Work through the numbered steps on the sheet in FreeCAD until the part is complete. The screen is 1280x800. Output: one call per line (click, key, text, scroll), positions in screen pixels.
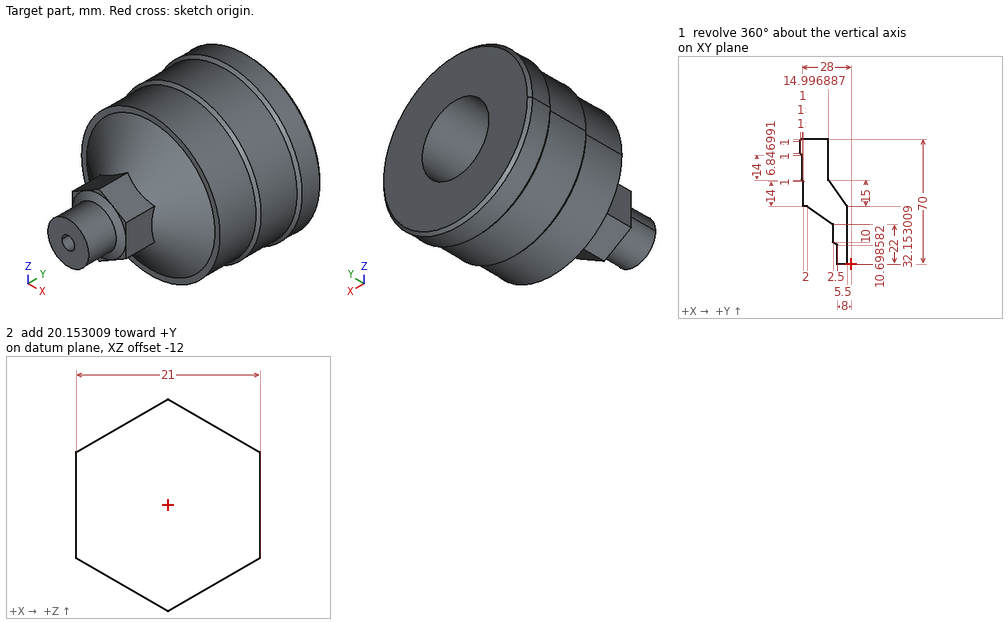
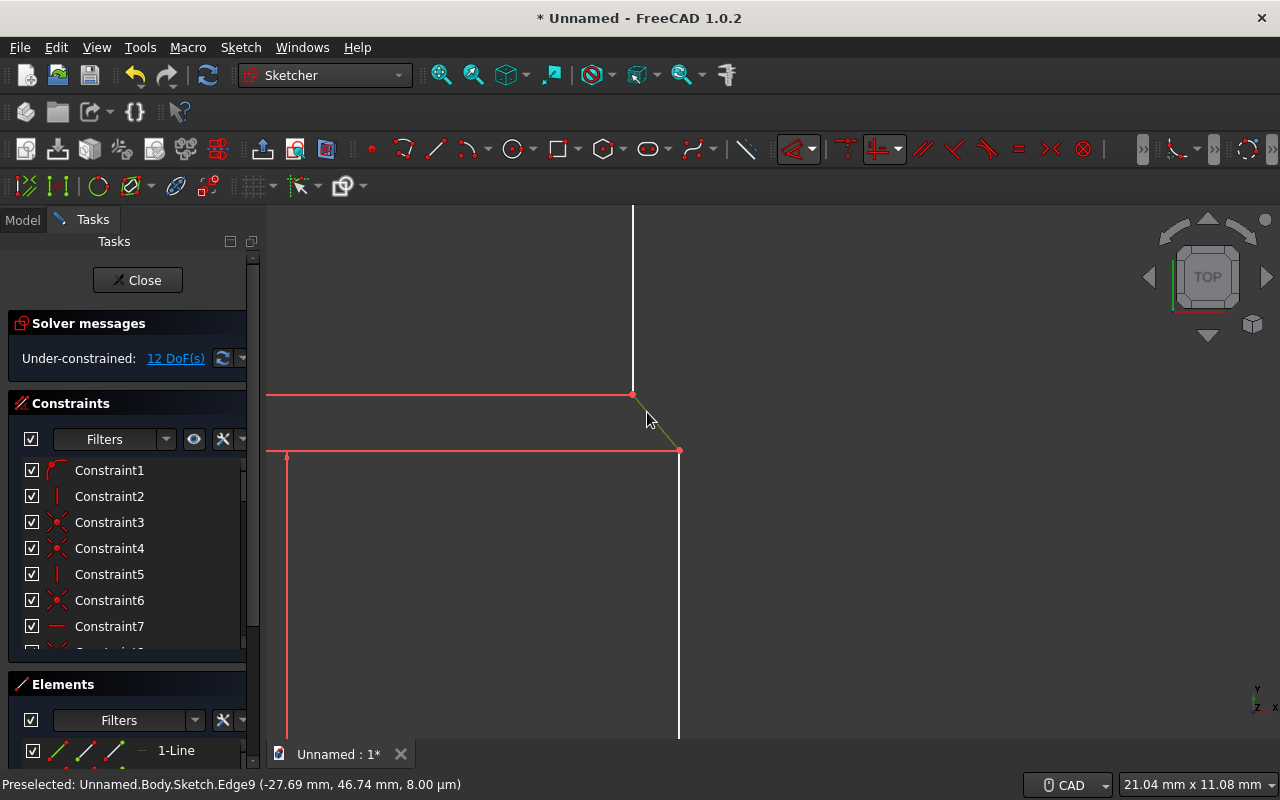
key(l)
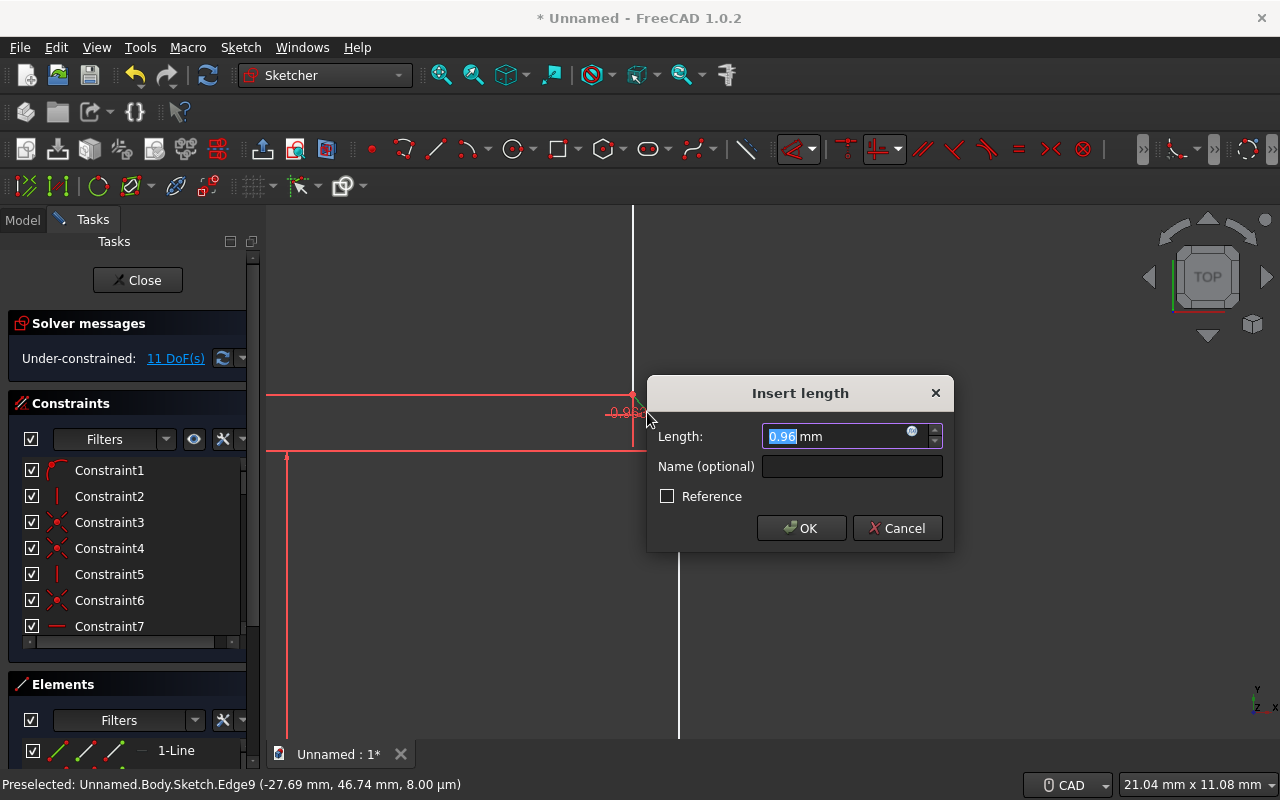
text(1)
key(Return)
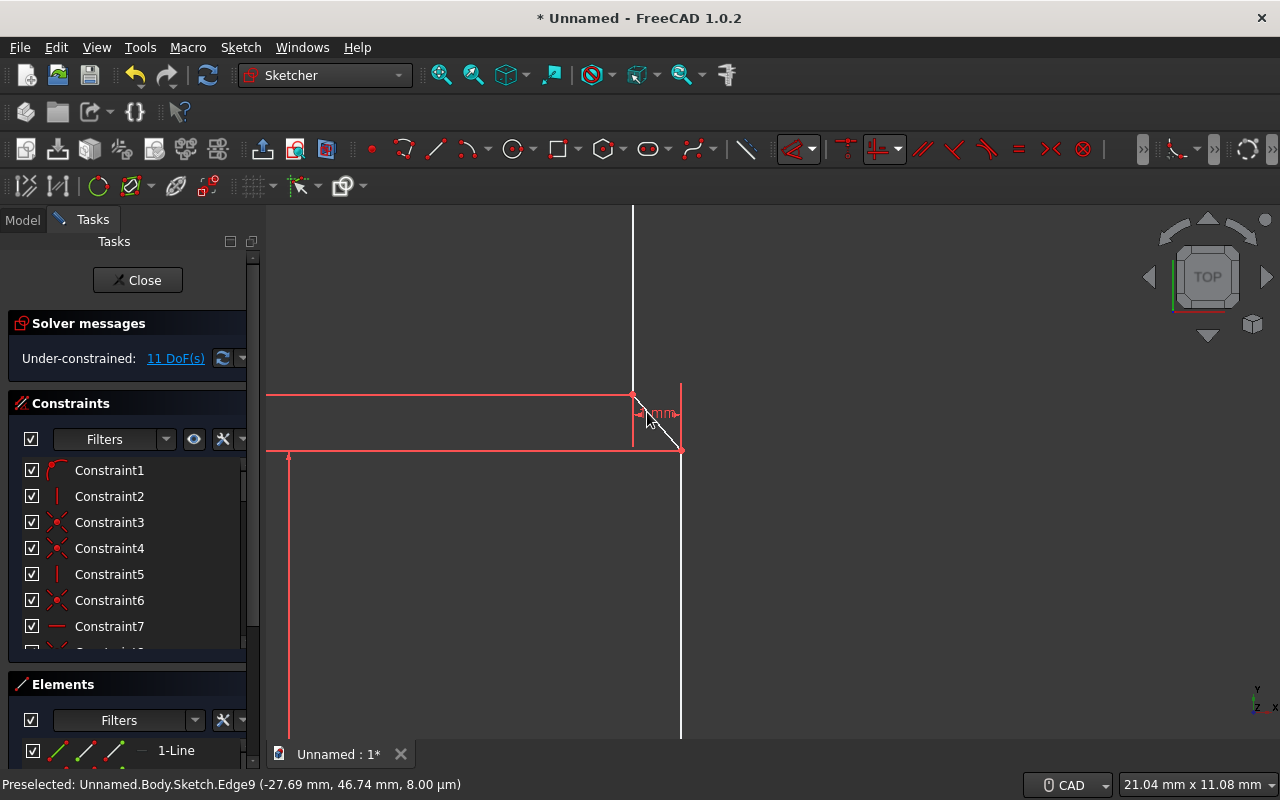
click(667, 434)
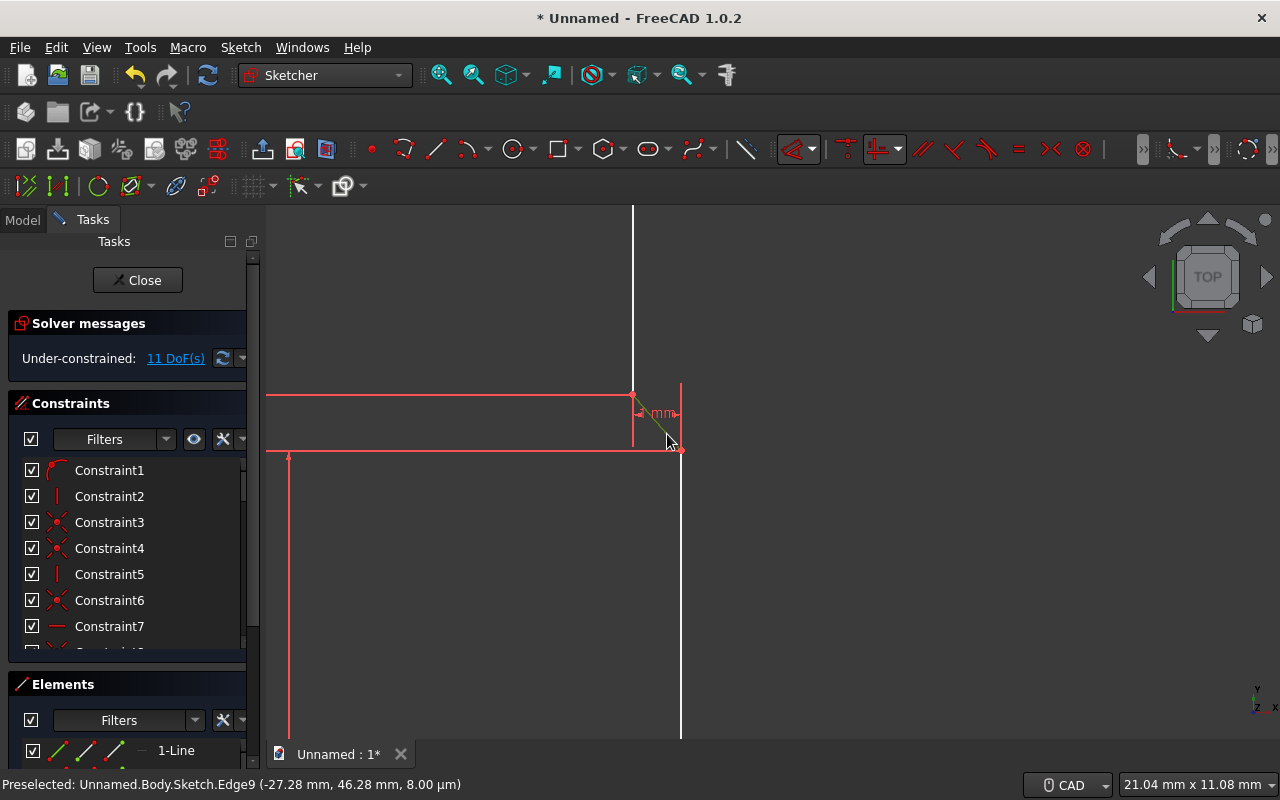
click(814, 150)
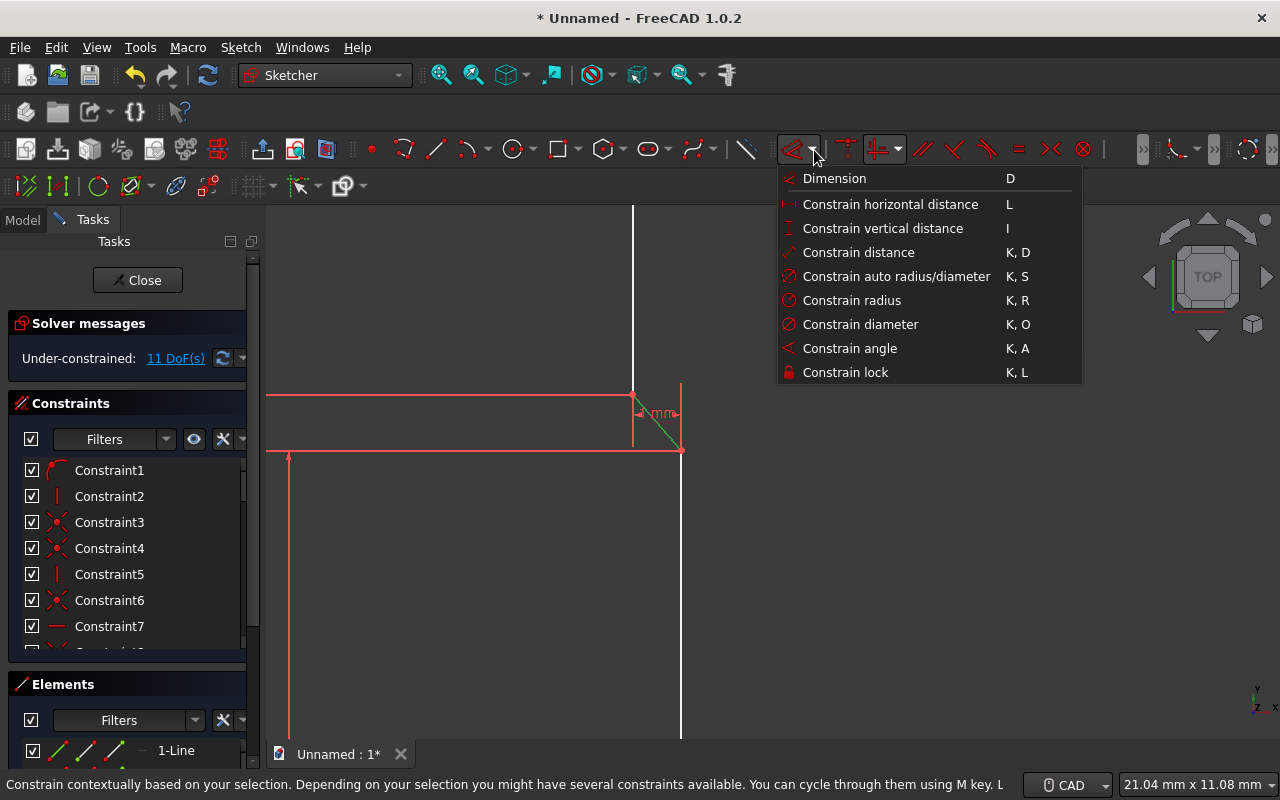
click(930, 228)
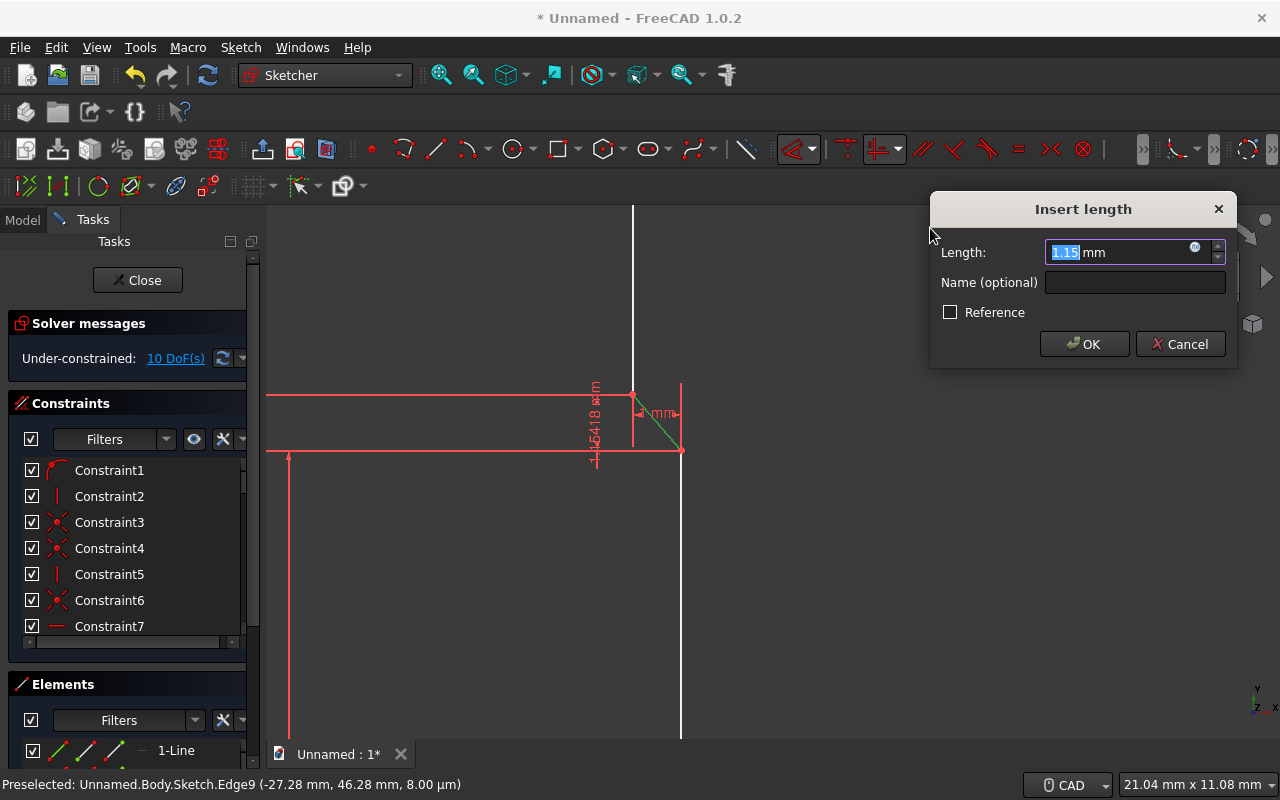
text(1)
key(Return)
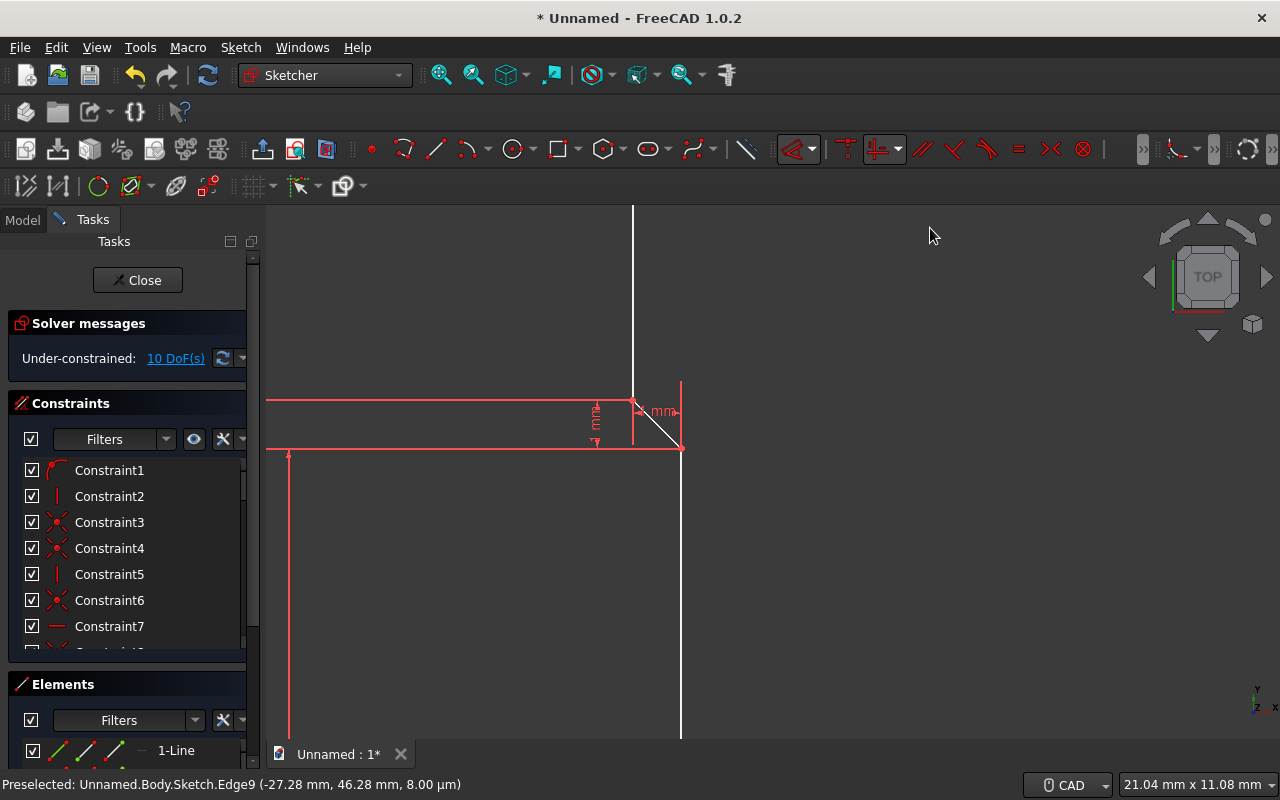
scroll(647, 422, down, 12)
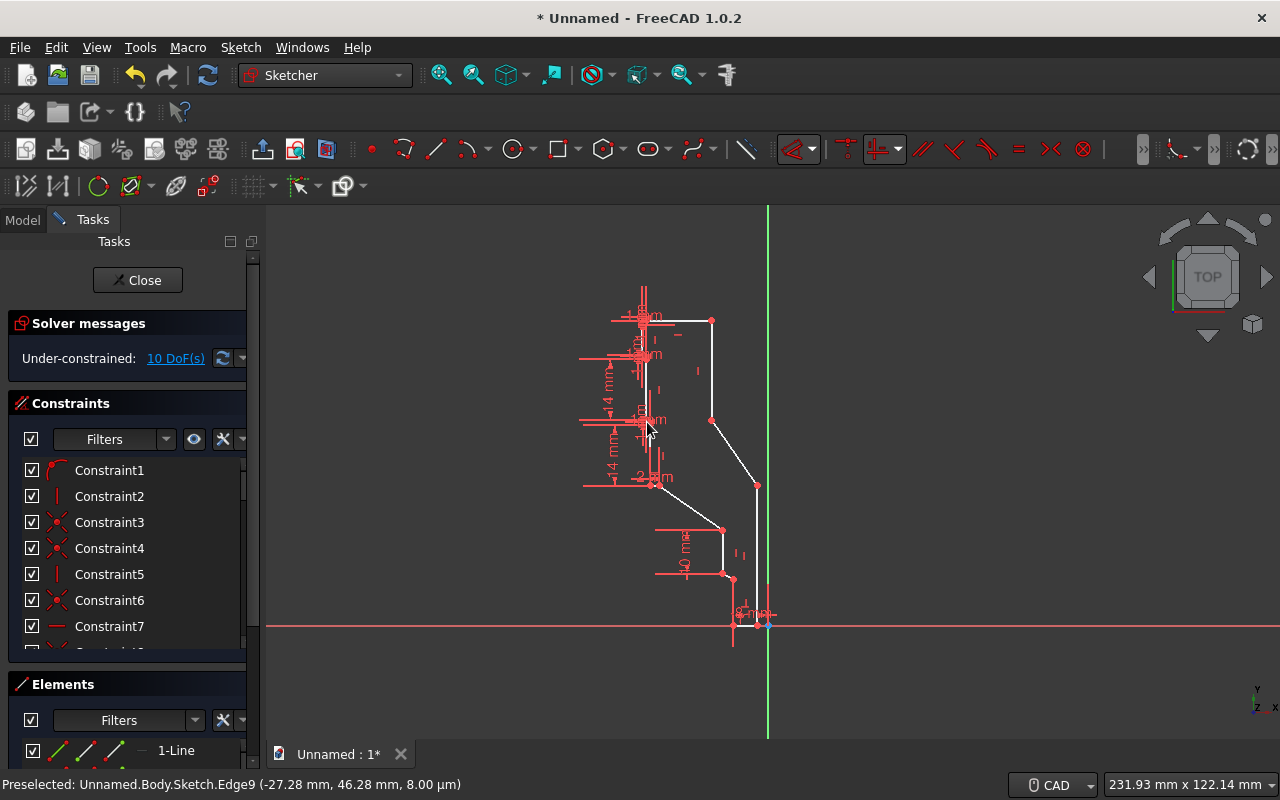
scroll(741, 626, up, 4)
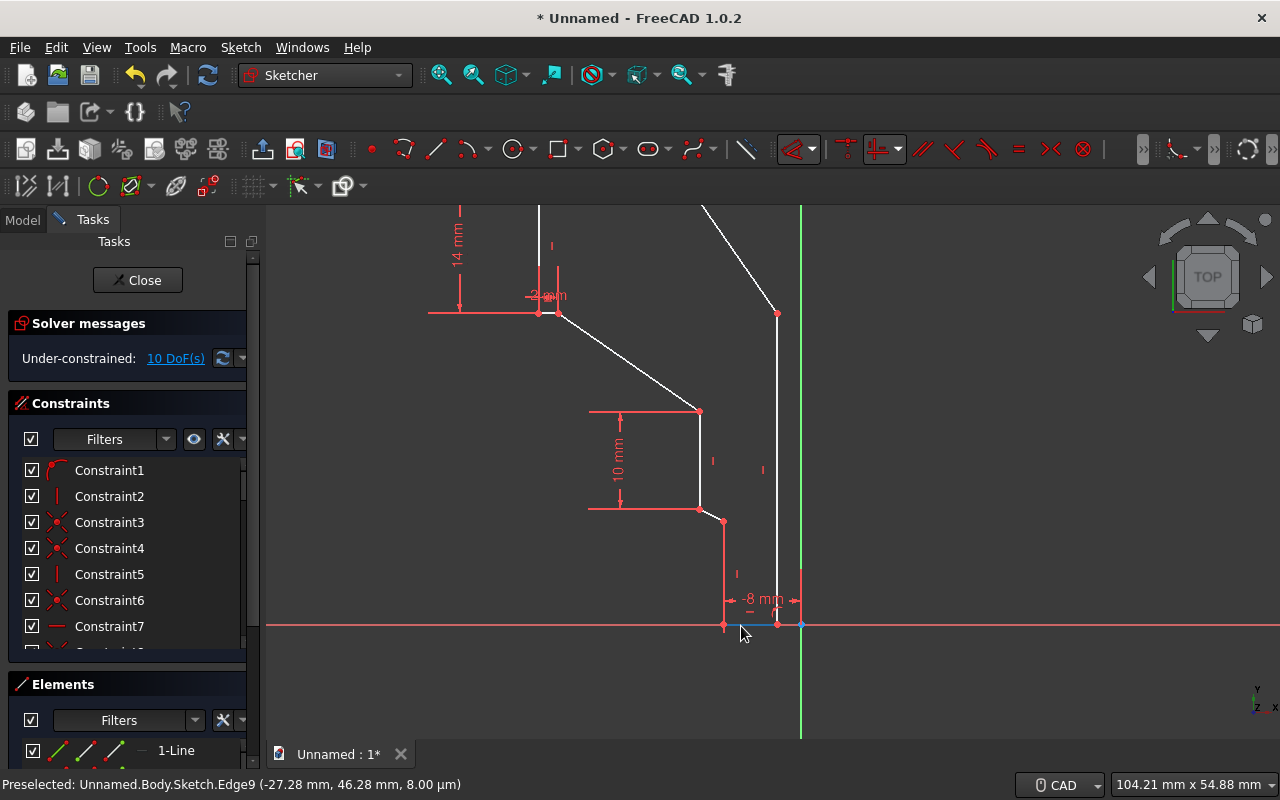
click(740, 625)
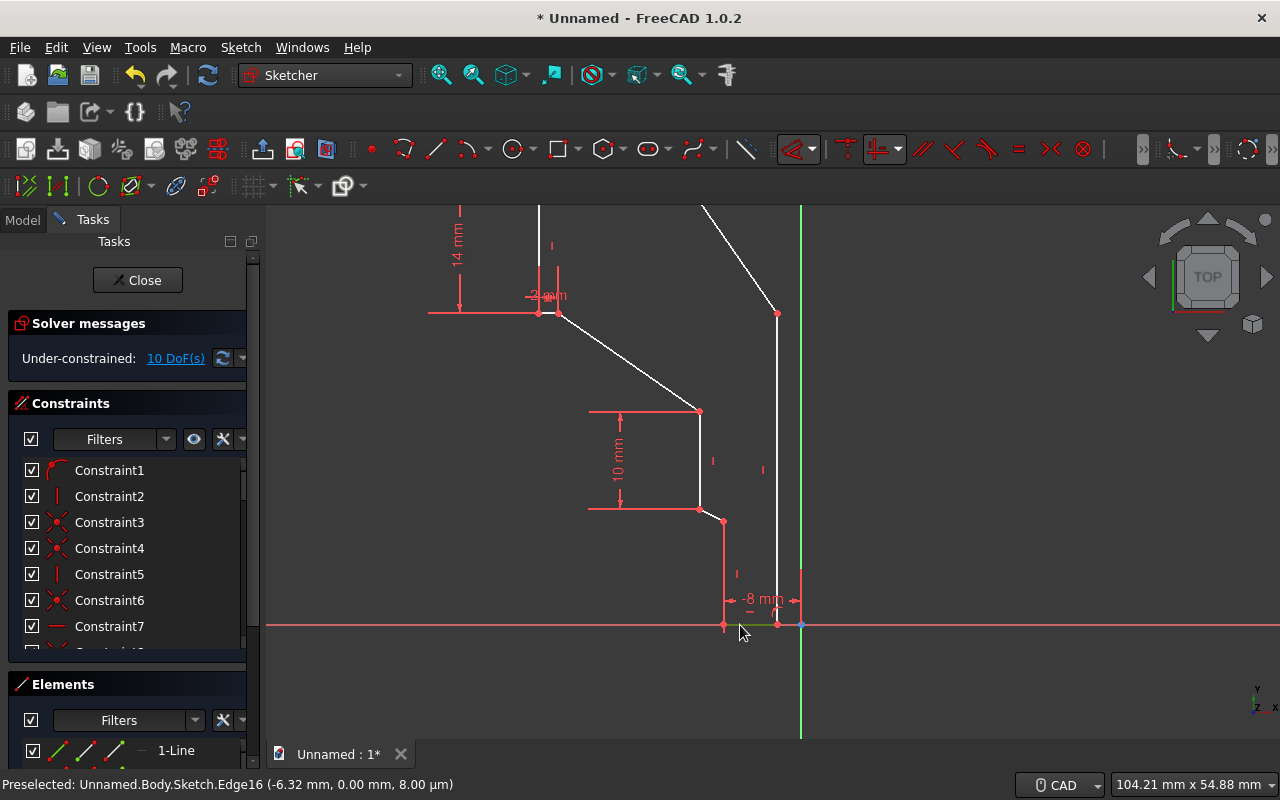
click(814, 150)